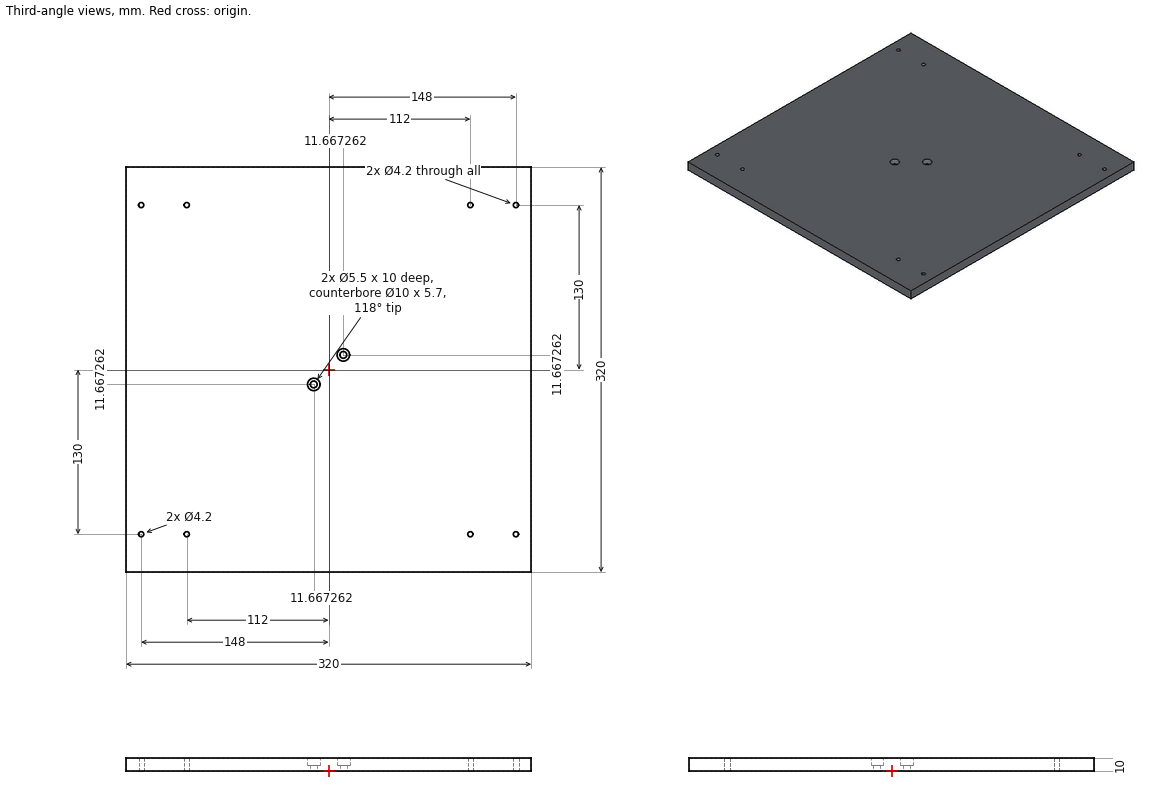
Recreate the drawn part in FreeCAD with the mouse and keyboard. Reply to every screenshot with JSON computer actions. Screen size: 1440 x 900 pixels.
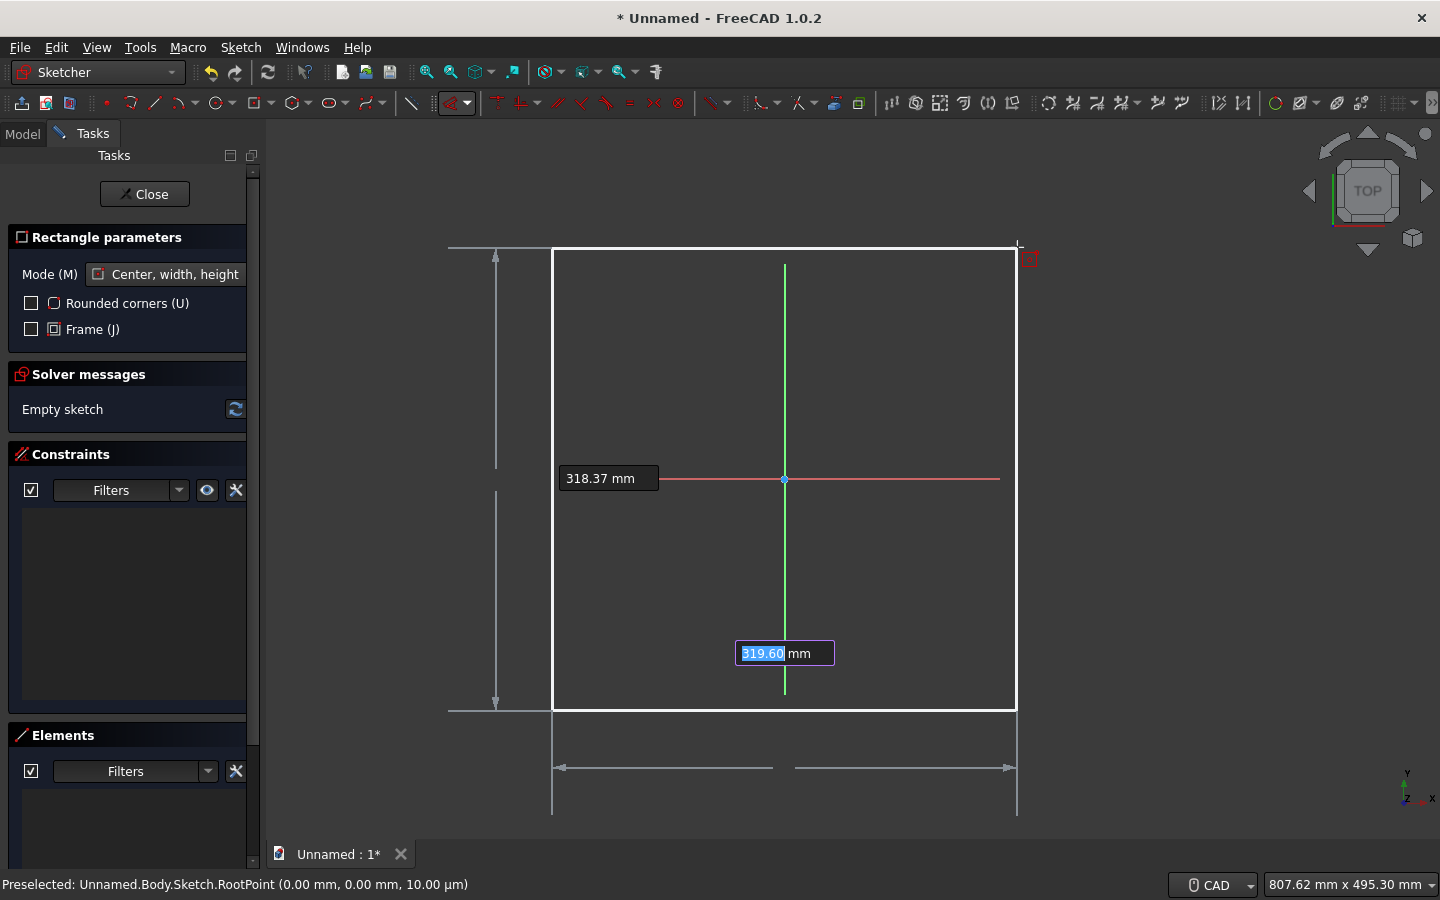
{"action": "type", "text": "320"}
{"action": "key", "text": "Tab"}
{"action": "type", "text": "320"}
{"action": "key", "text": "Return"}
{"action": "key", "text": "Escape"}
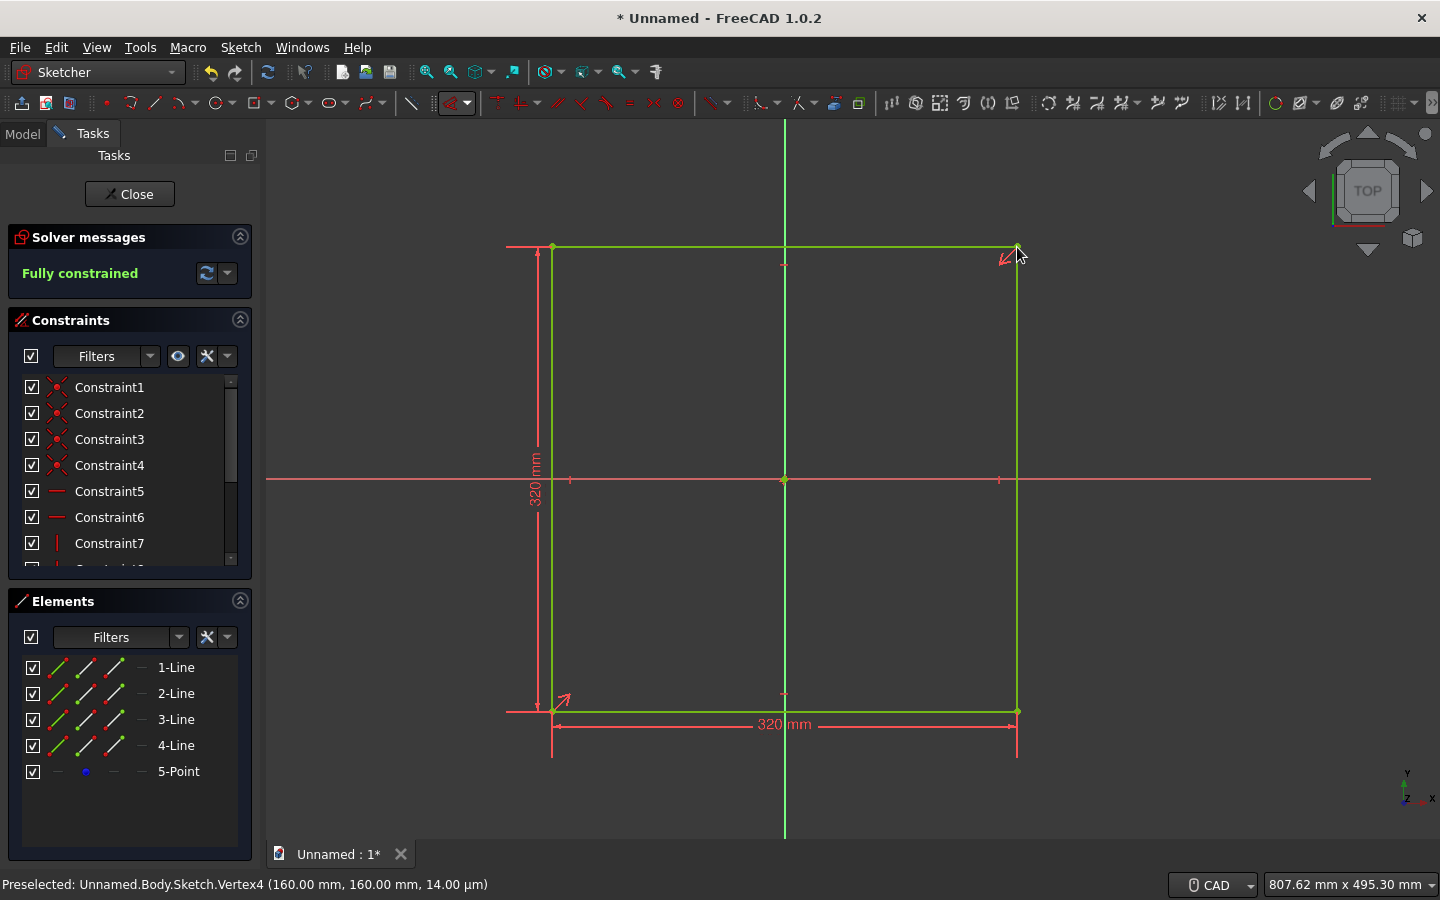
{"action": "left_click", "coordinate": [130, 194]}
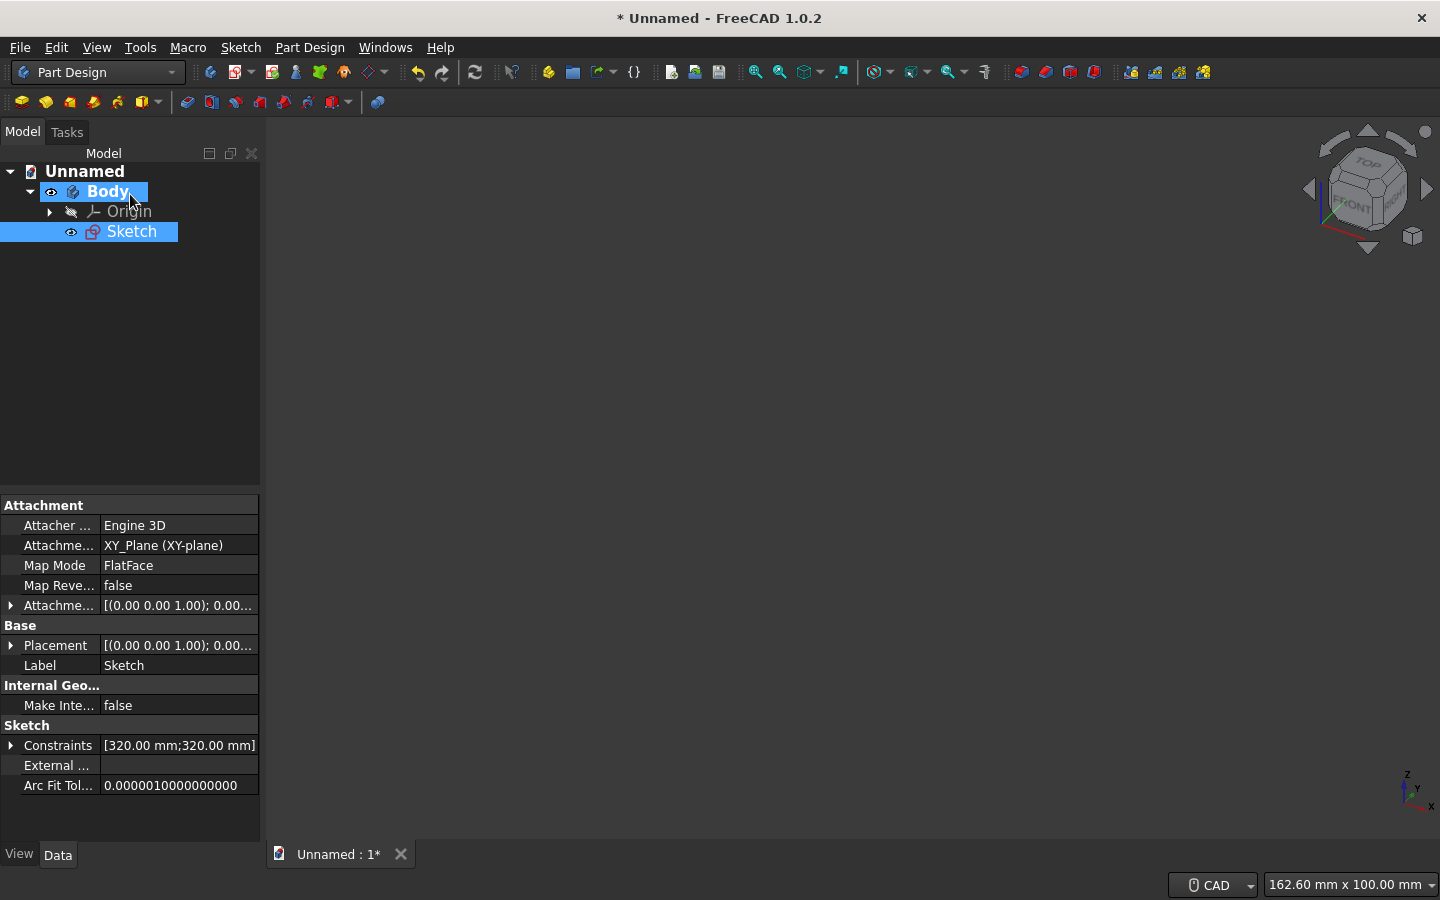
{"action": "left_click", "coordinate": [22, 102]}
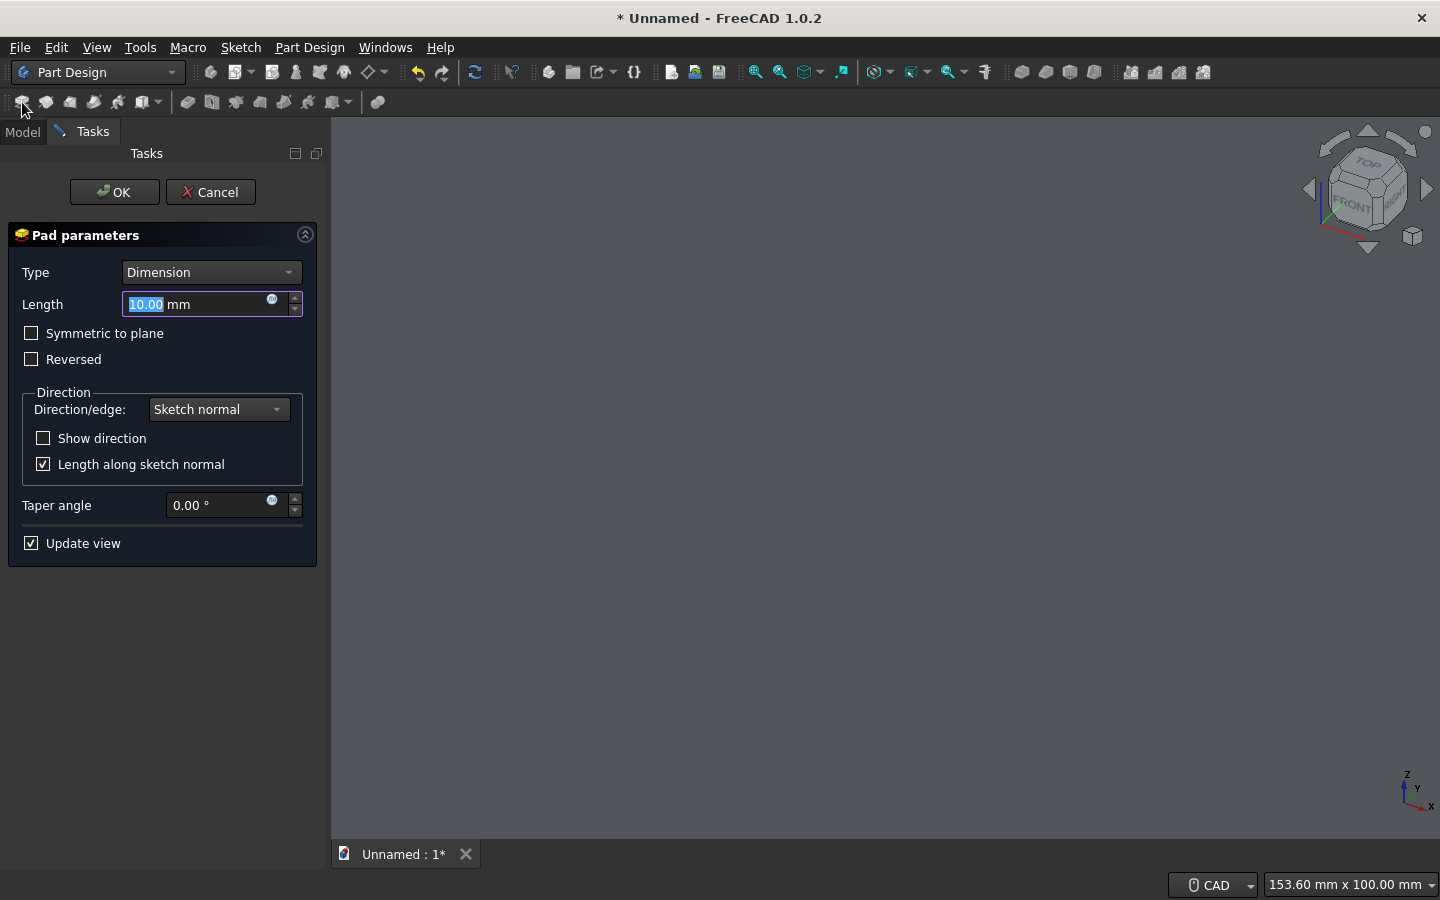
{"action": "type", "text": "10"}
{"action": "key", "text": "Tab"}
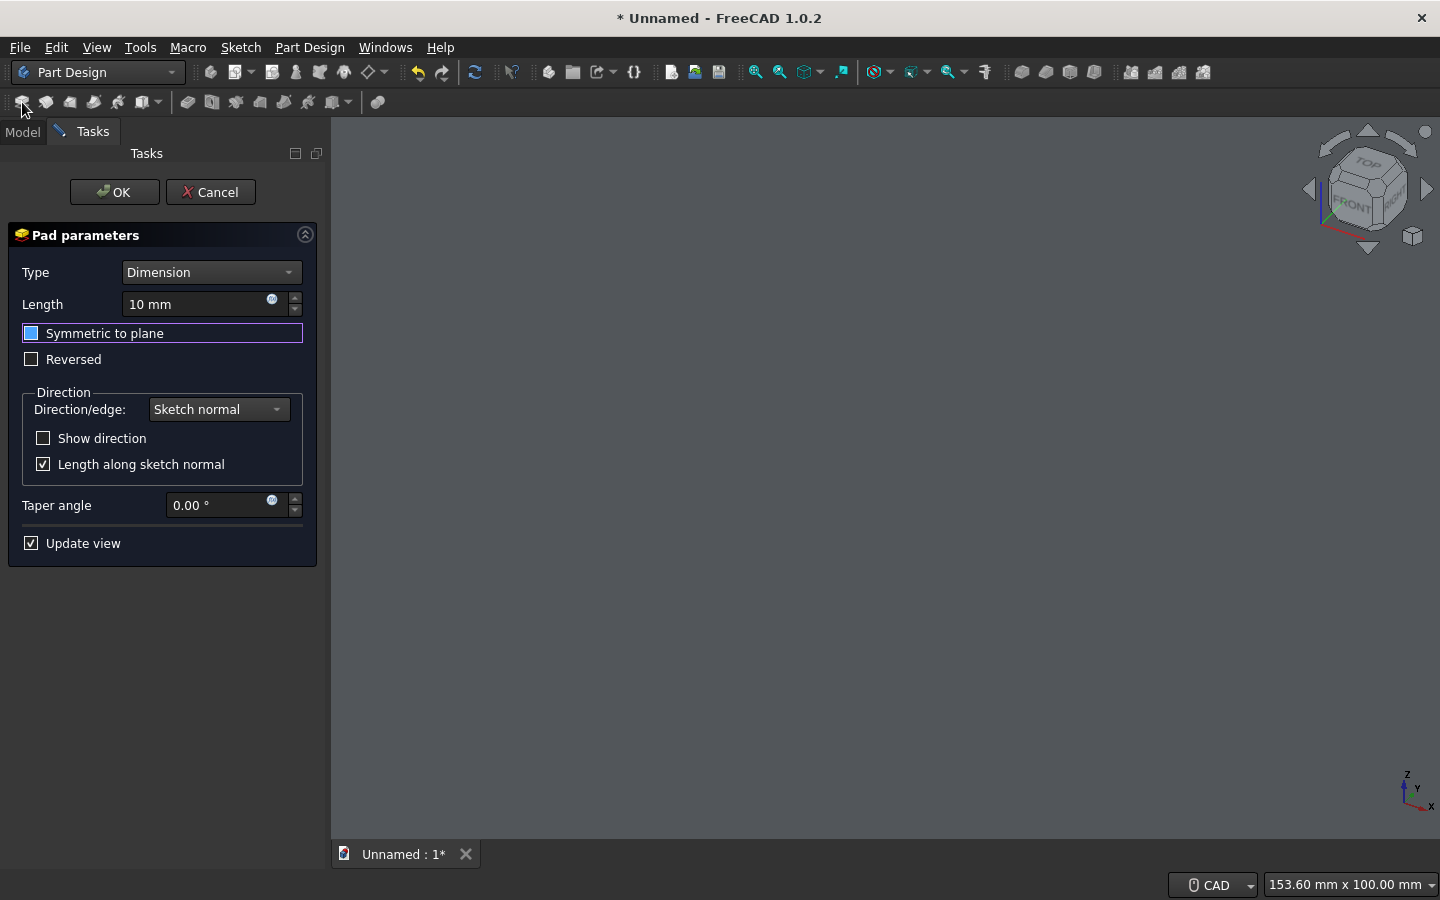
{"action": "left_click", "coordinate": [115, 192]}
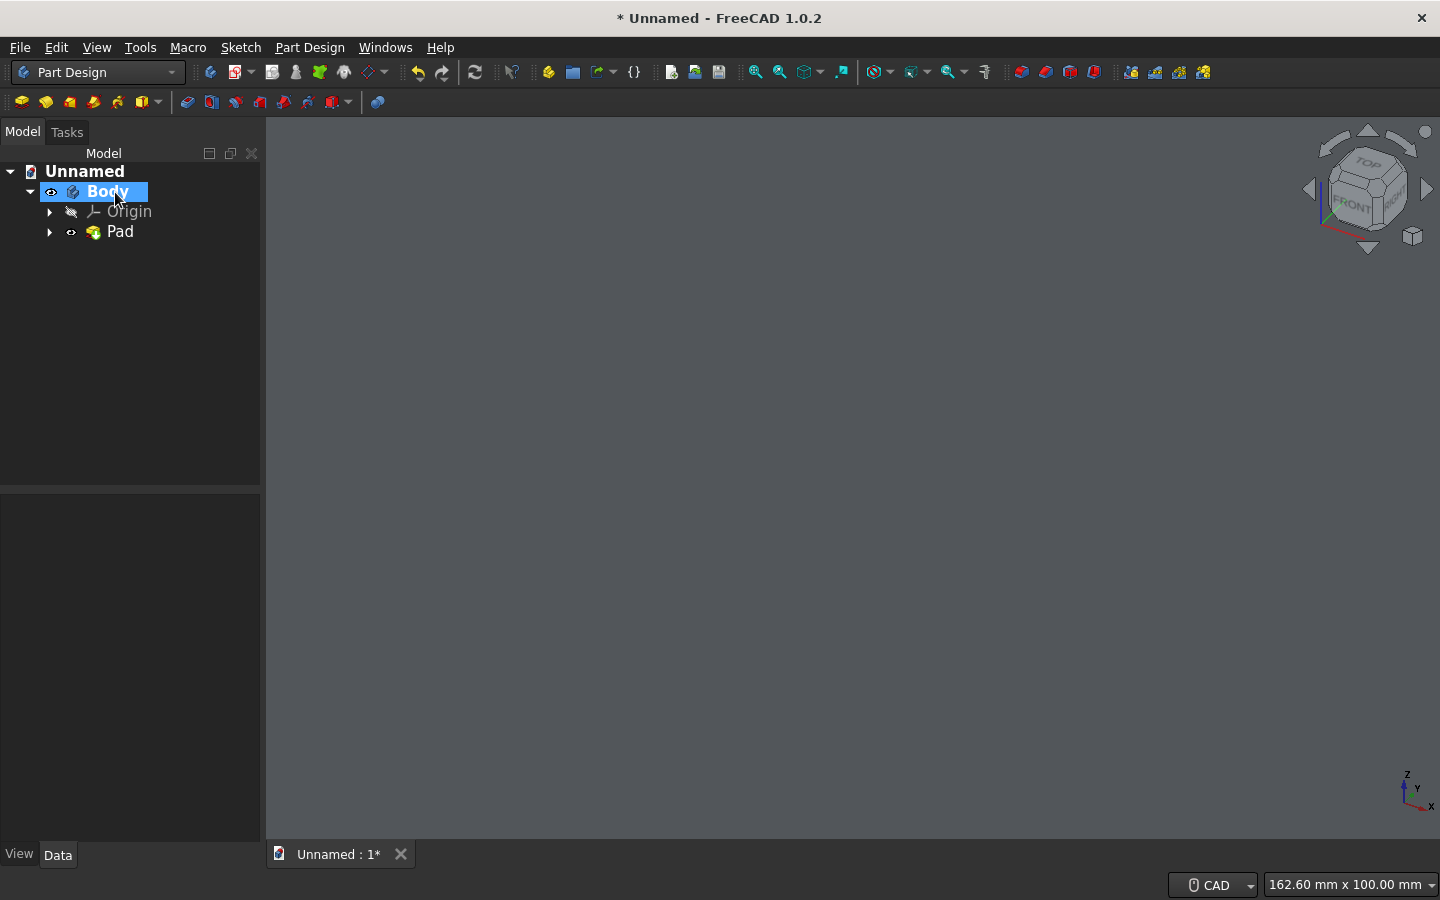
{"action": "key", "text": "v f"}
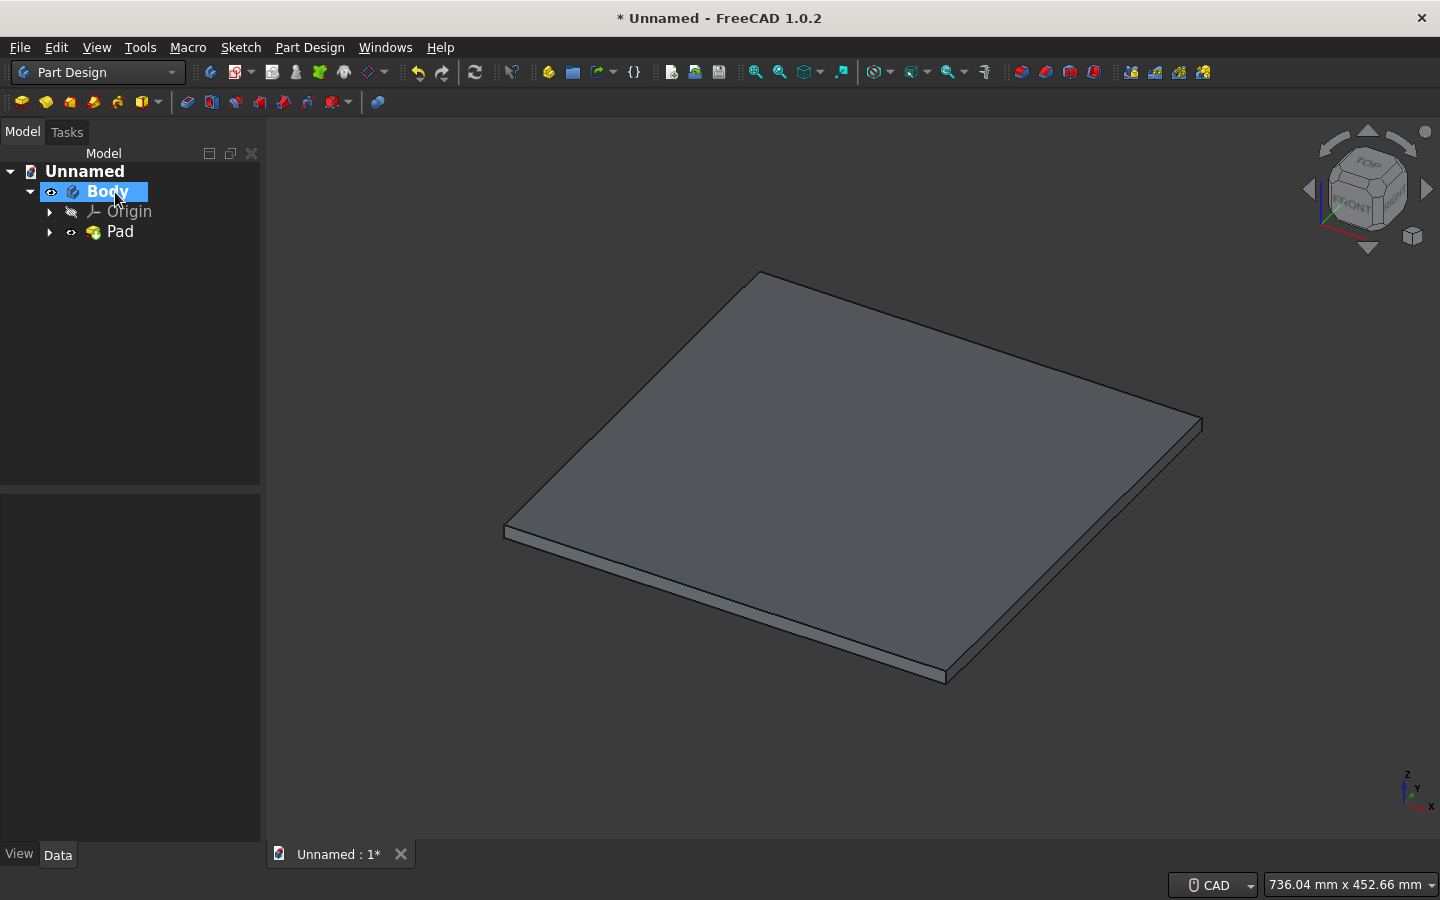
{"action": "left_click", "coordinate": [853, 470]}